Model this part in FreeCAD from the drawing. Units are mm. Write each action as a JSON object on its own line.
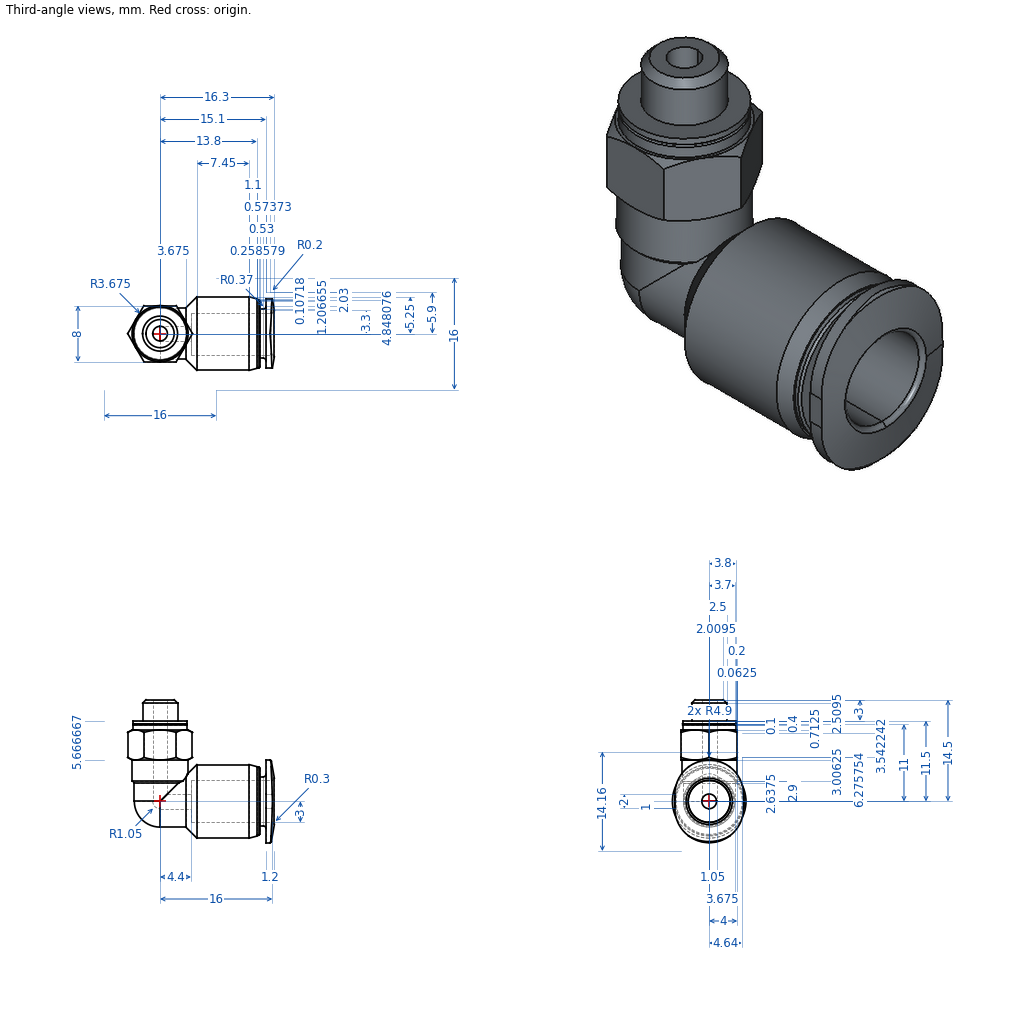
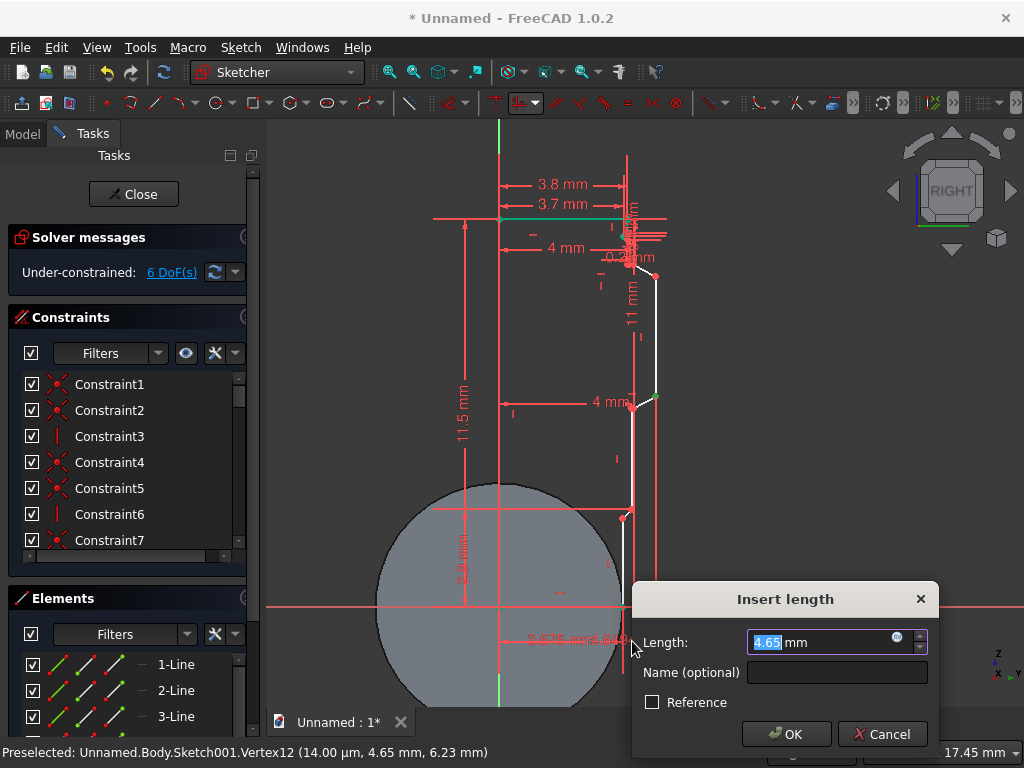
{"action": "type", "text": "4.64"}
{"action": "key", "text": "Return"}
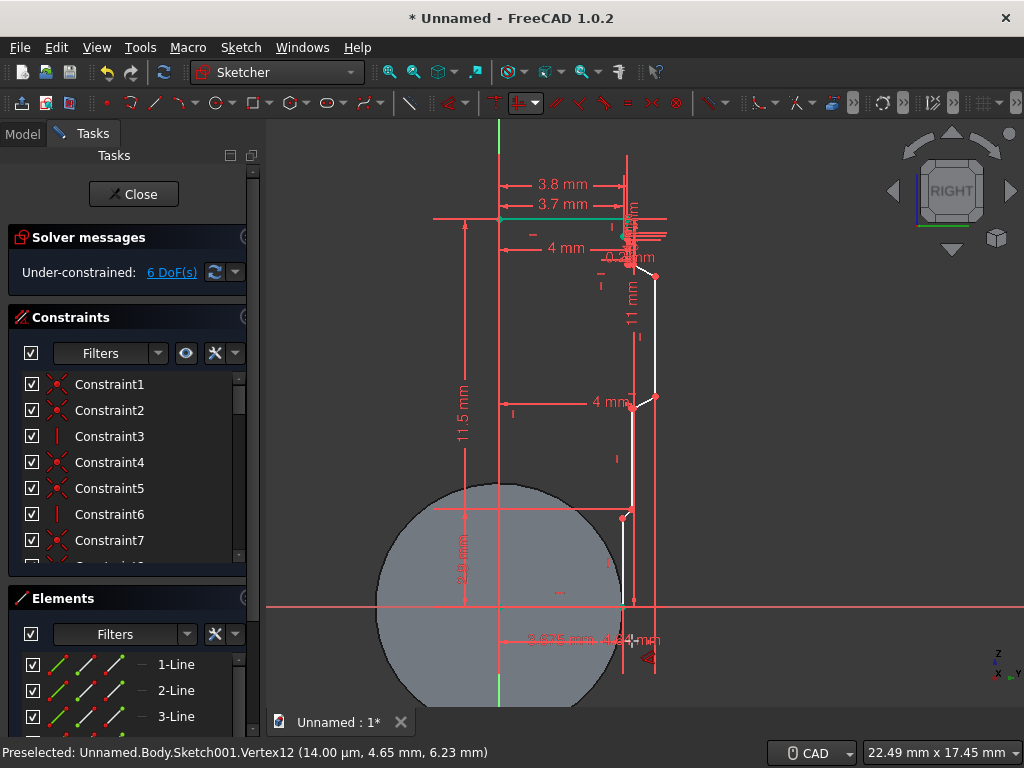
{"action": "left_click", "coordinate": [623, 581]}
{"action": "left_click", "coordinate": [657, 563]}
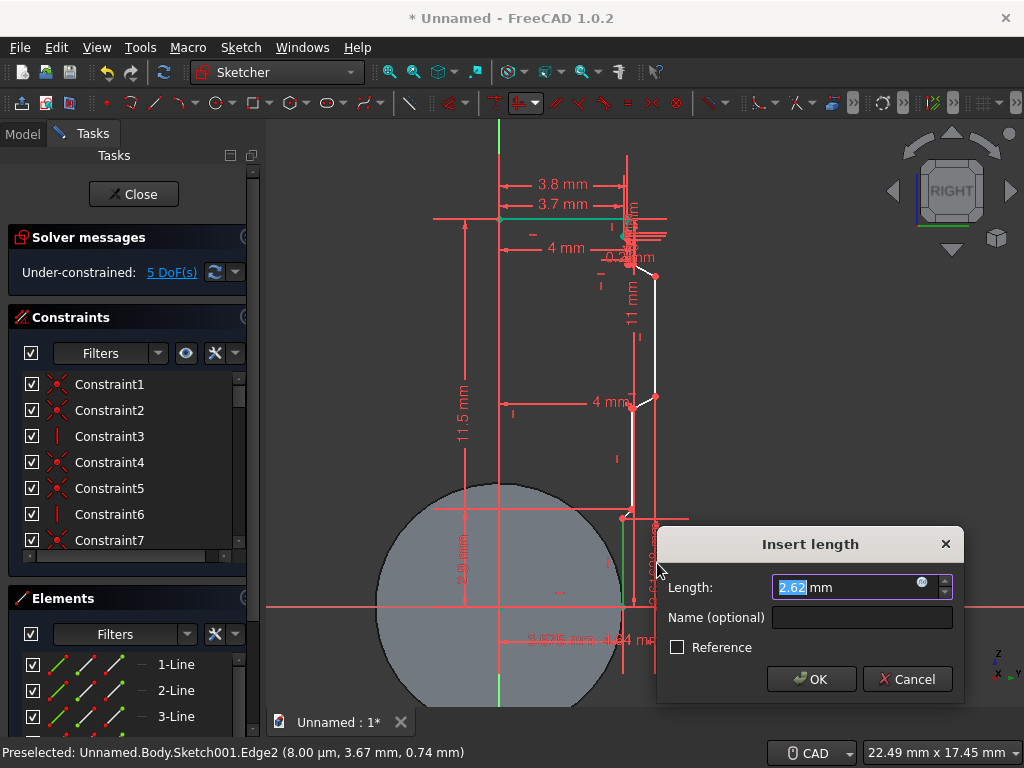
{"action": "type", "text": "2.6375"}
{"action": "key", "text": "Return"}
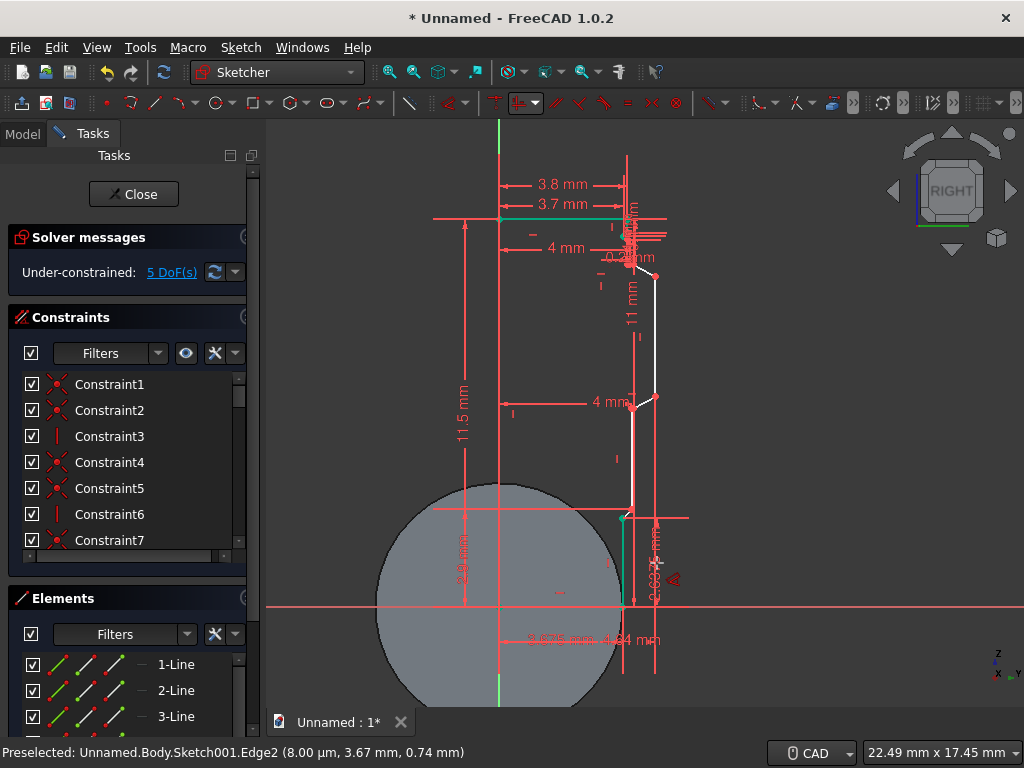
{"action": "scroll", "coordinate": [633, 409], "scroll_direction": "up", "scroll_amount": 15}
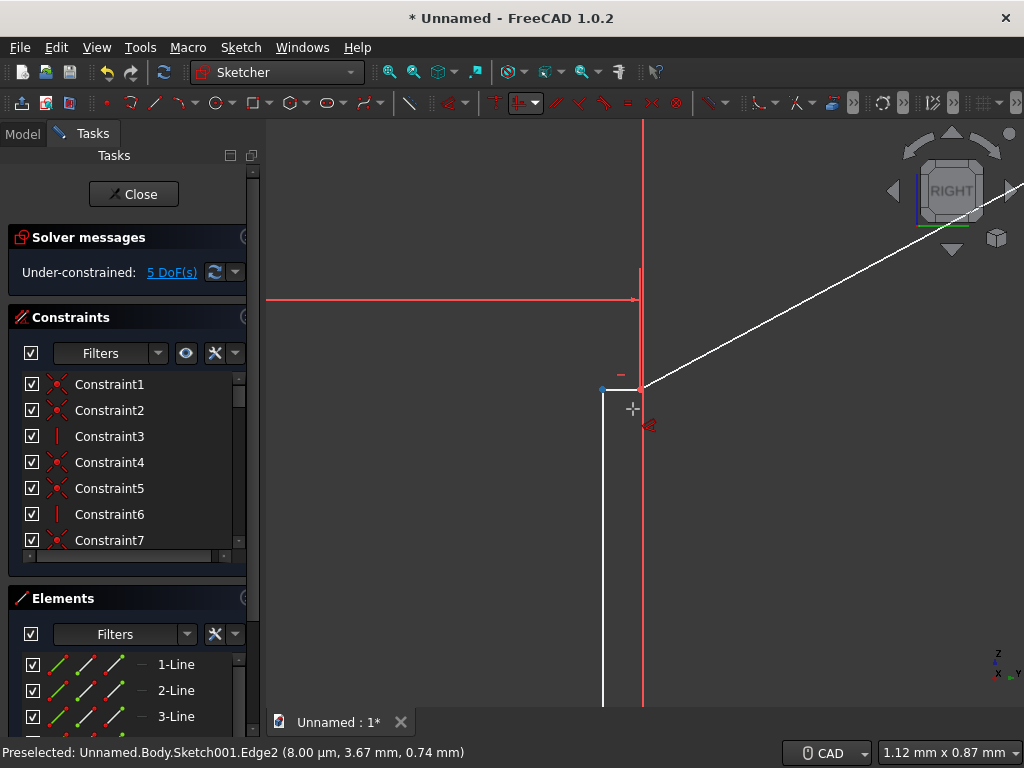
{"action": "left_click", "coordinate": [622, 390]}
{"action": "left_click", "coordinate": [622, 356]}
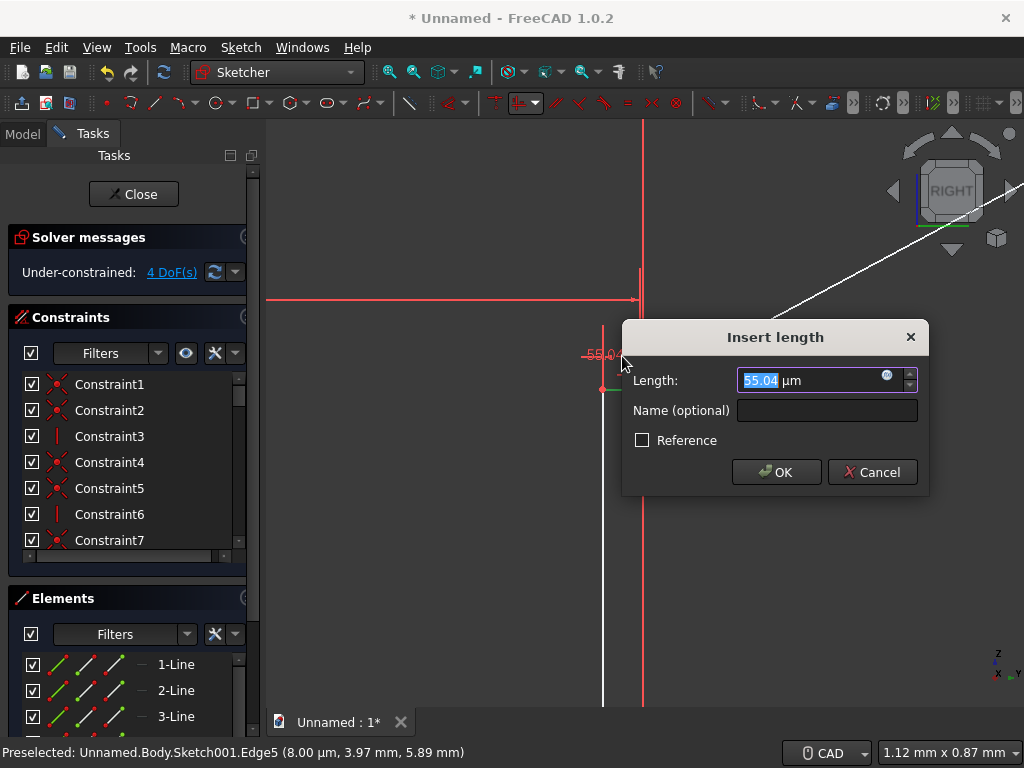
{"action": "key", "text": "ctrl+a"}
{"action": "type", "text": "0.0625 mm"}
{"action": "key", "text": "Return"}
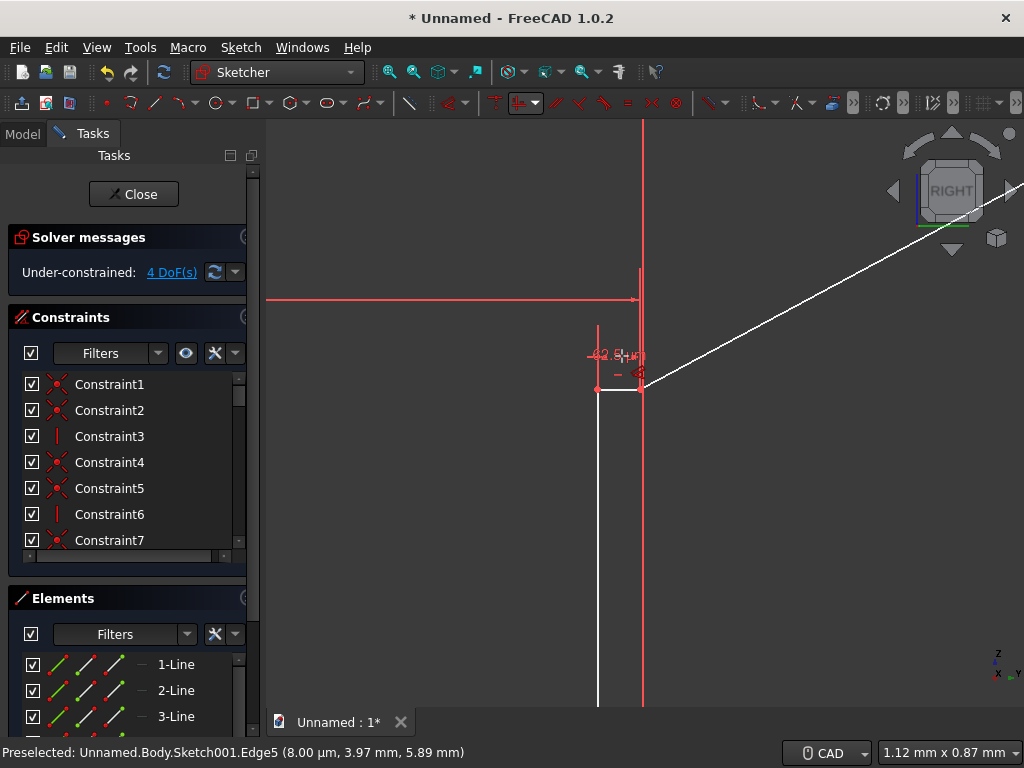
{"action": "scroll", "coordinate": [633, 409], "scroll_direction": "down", "scroll_amount": 15}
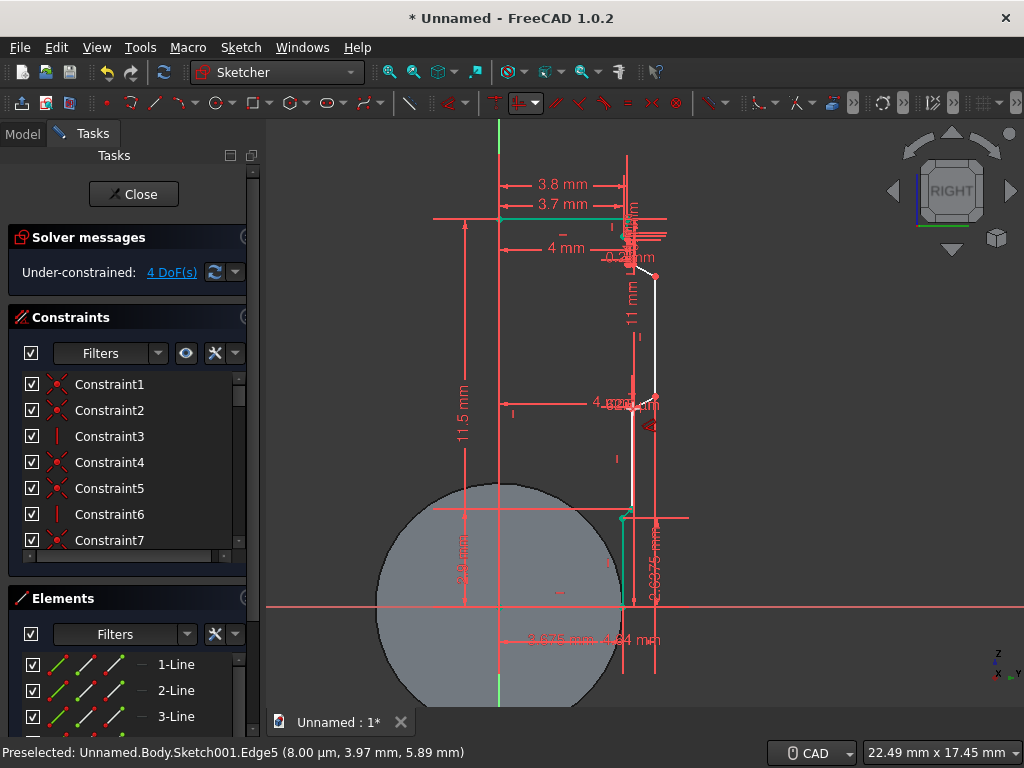
{"action": "scroll", "coordinate": [627, 257], "scroll_direction": "up", "scroll_amount": 3}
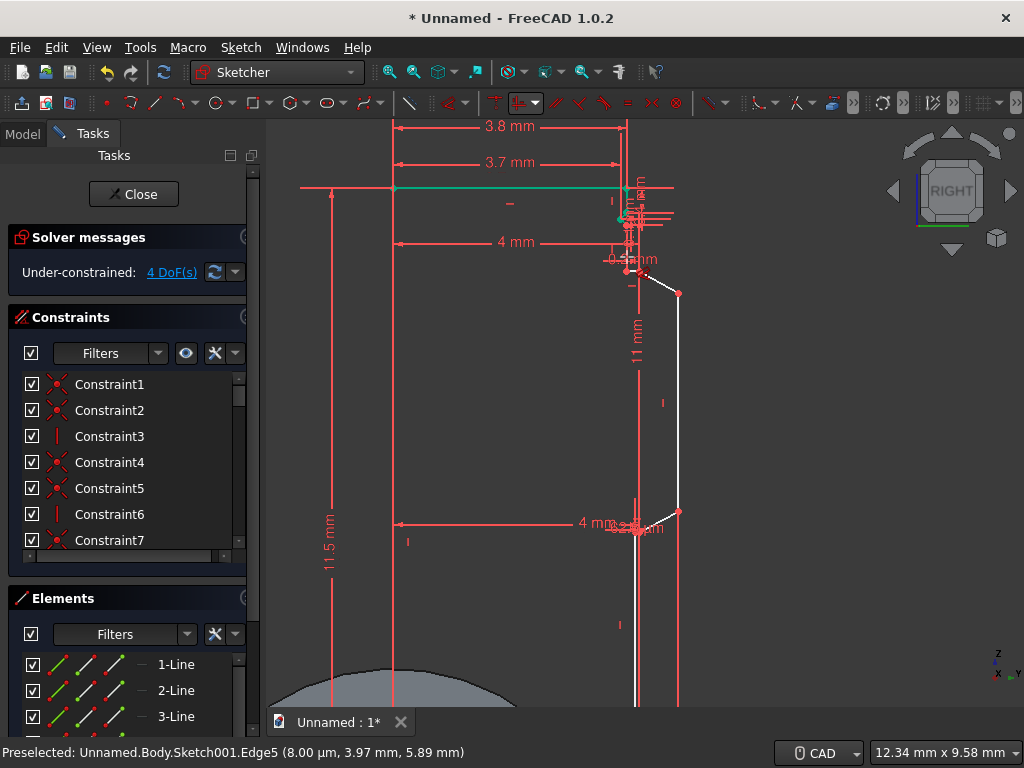
{"action": "left_click", "coordinate": [627, 257]}
{"action": "left_click", "coordinate": [709, 248]}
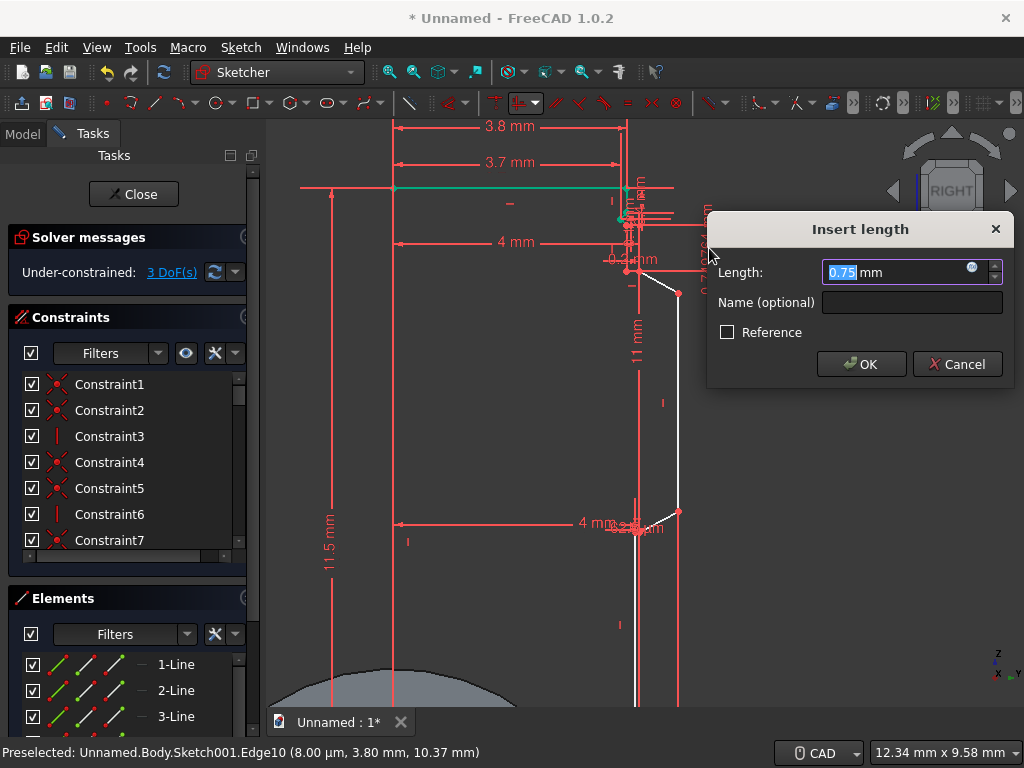
{"action": "type", "text": "0.7125"}
{"action": "key", "text": "Return"}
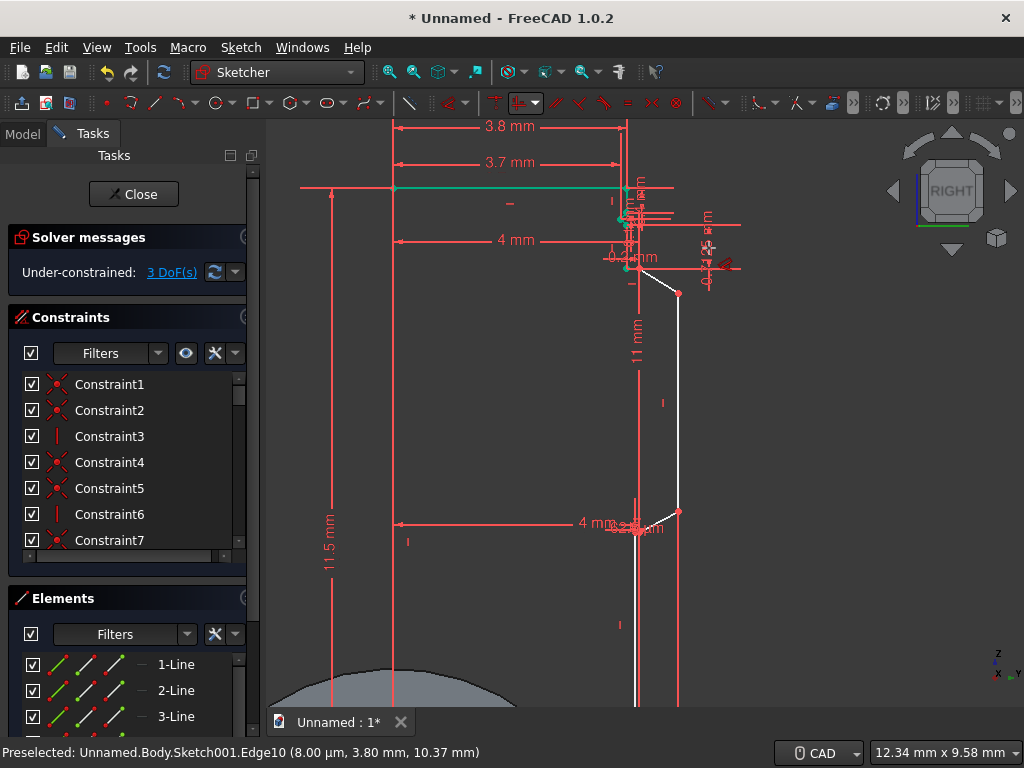
{"action": "left_click", "coordinate": [635, 661]}
{"action": "left_click", "coordinate": [669, 606]}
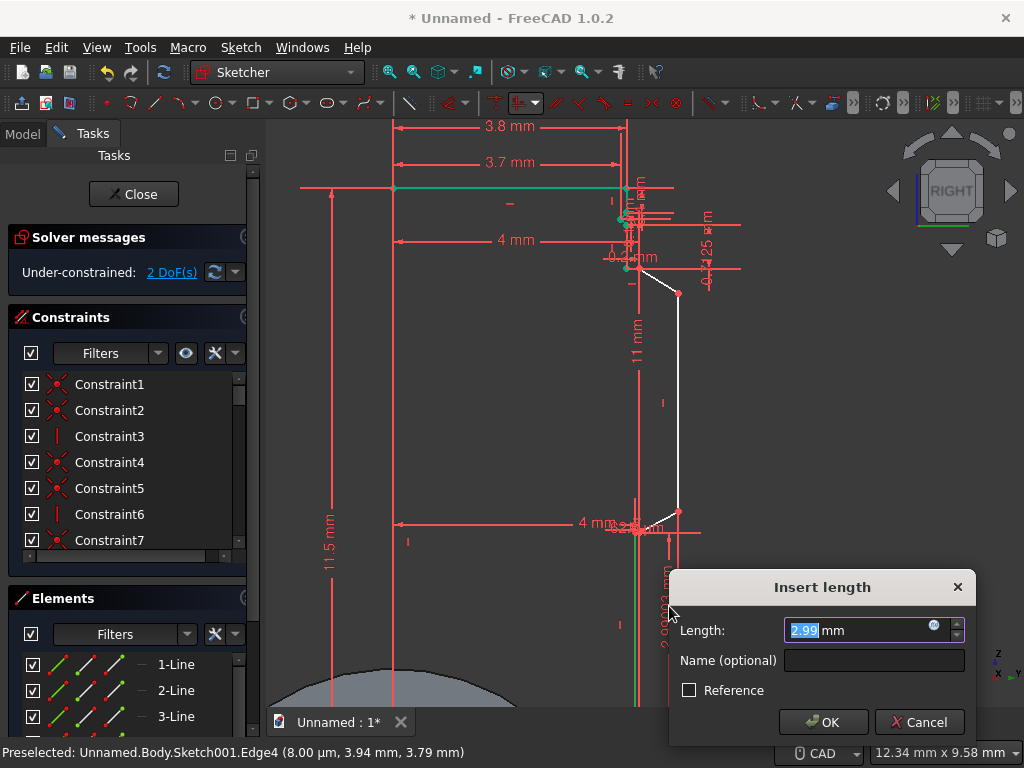
{"action": "type", "text": "3.00625"}
{"action": "key", "text": "Return"}